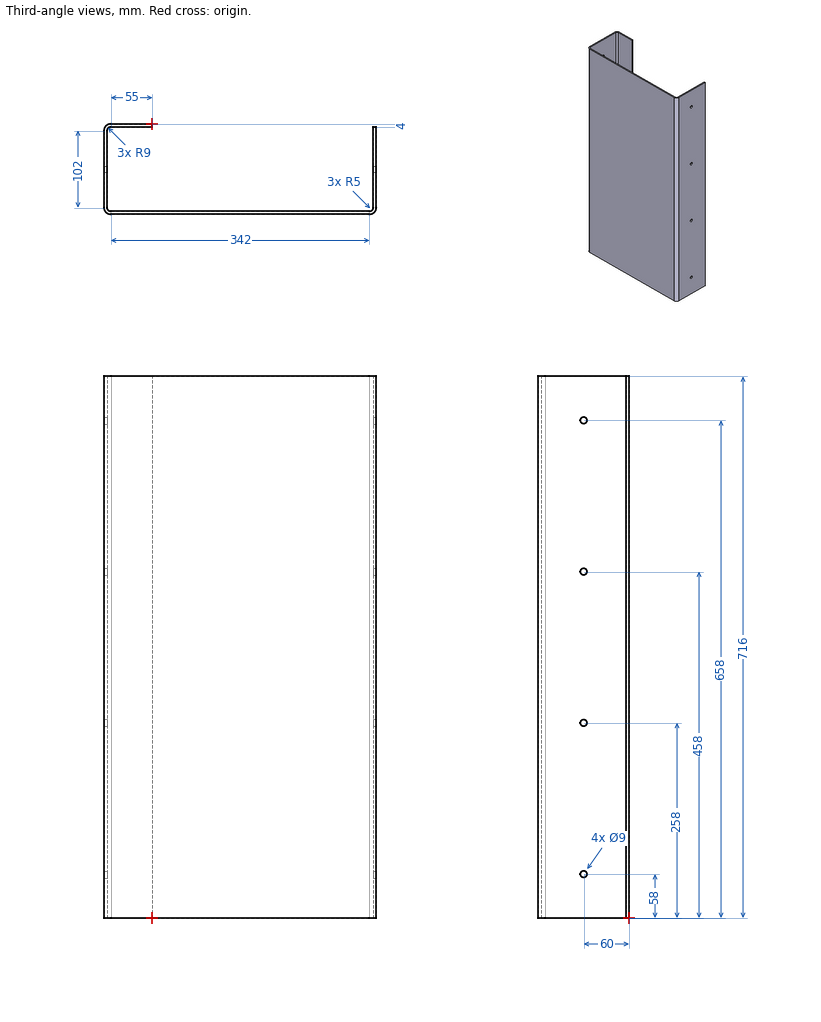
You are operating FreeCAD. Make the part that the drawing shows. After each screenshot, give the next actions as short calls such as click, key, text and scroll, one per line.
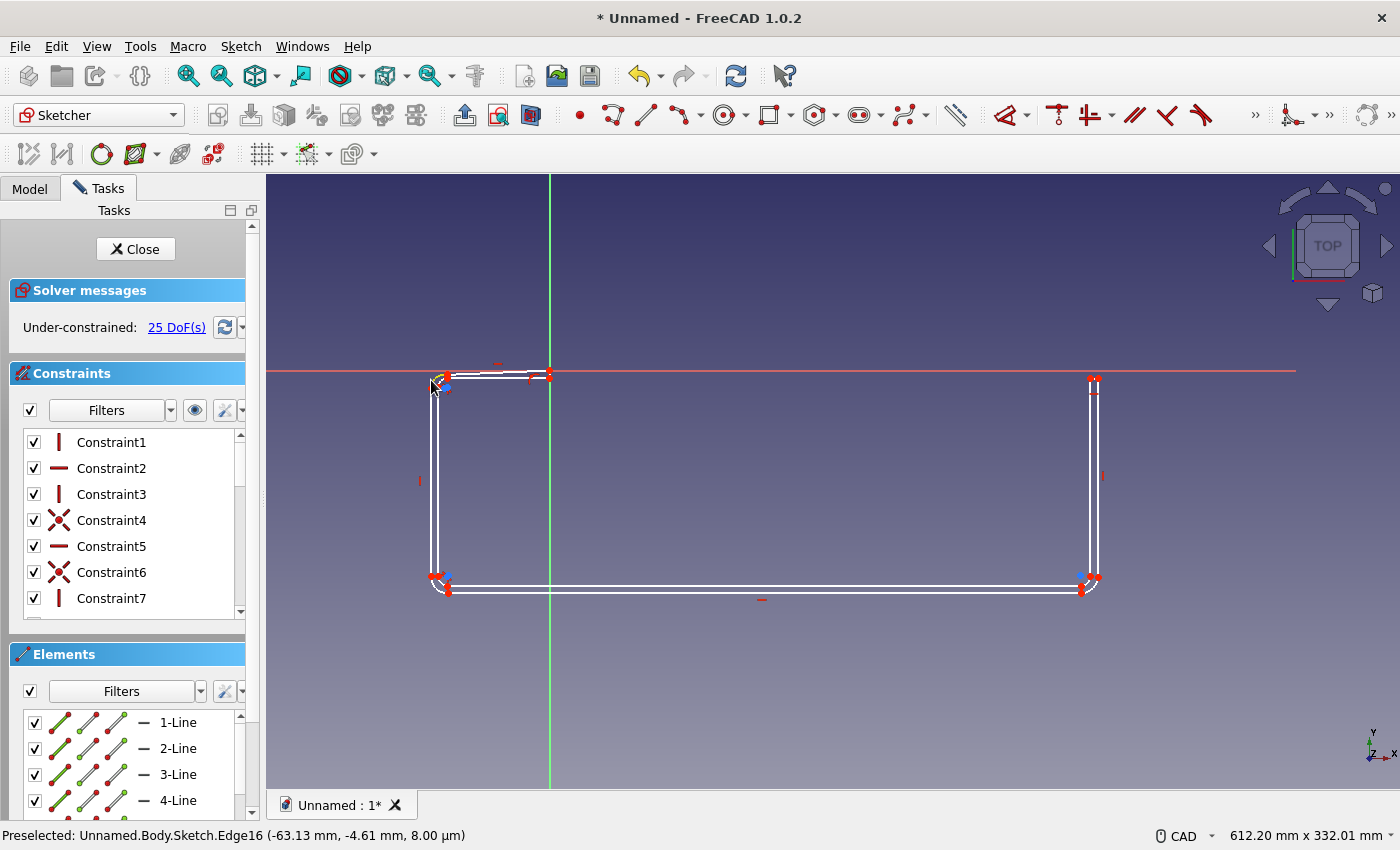
scroll(638, 593, up, 4)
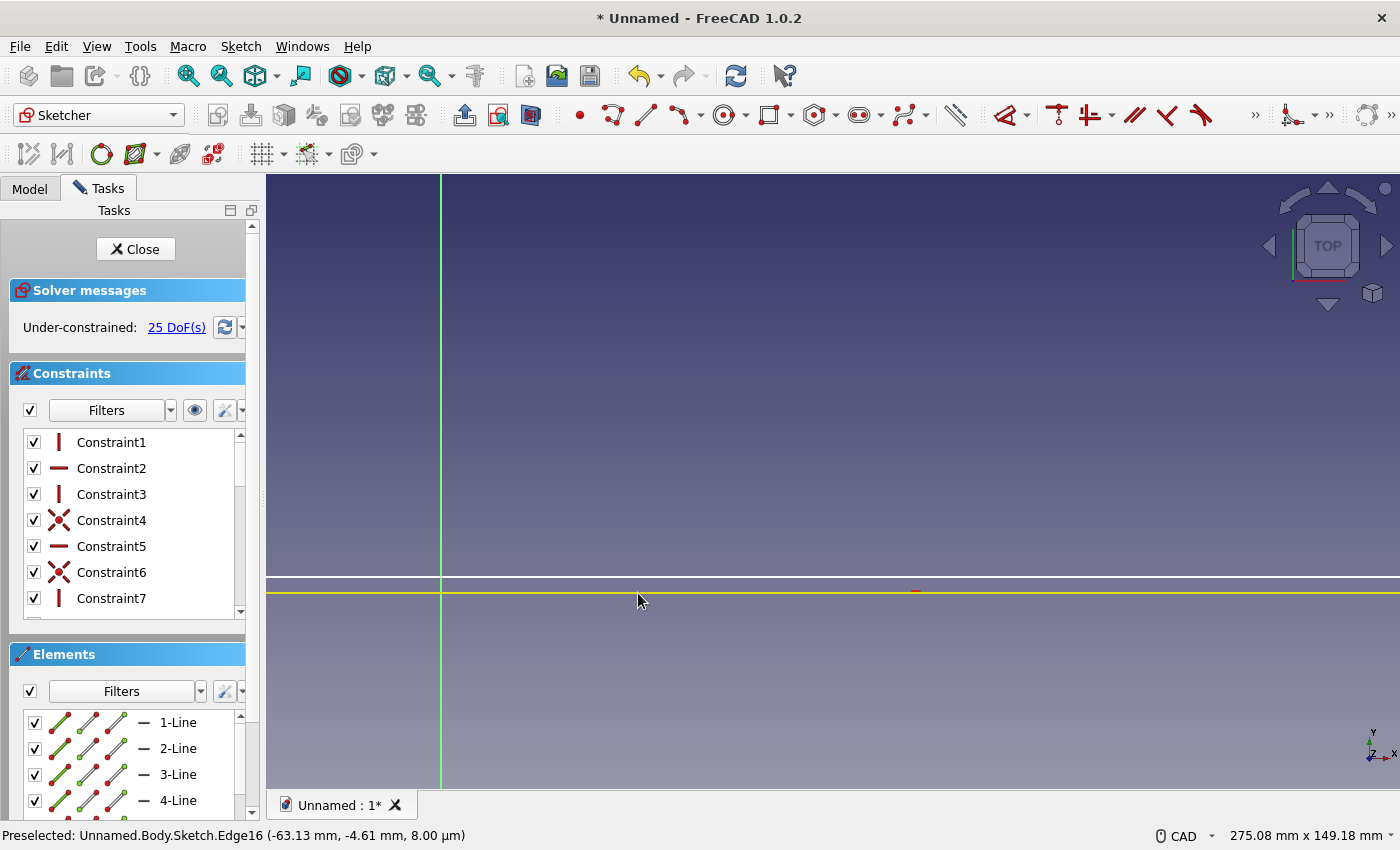
click(638, 593)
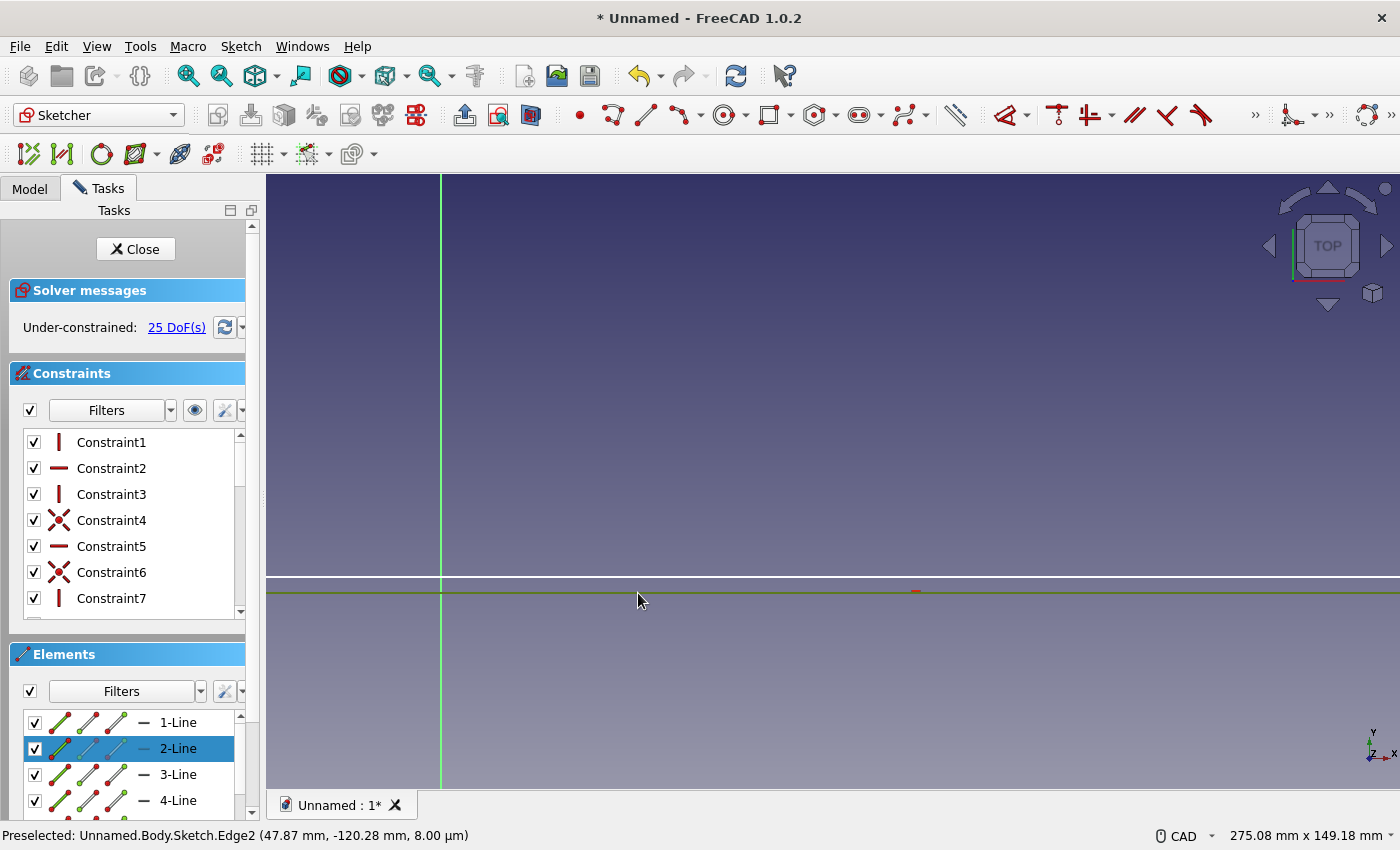
scroll(639, 593, down, 4)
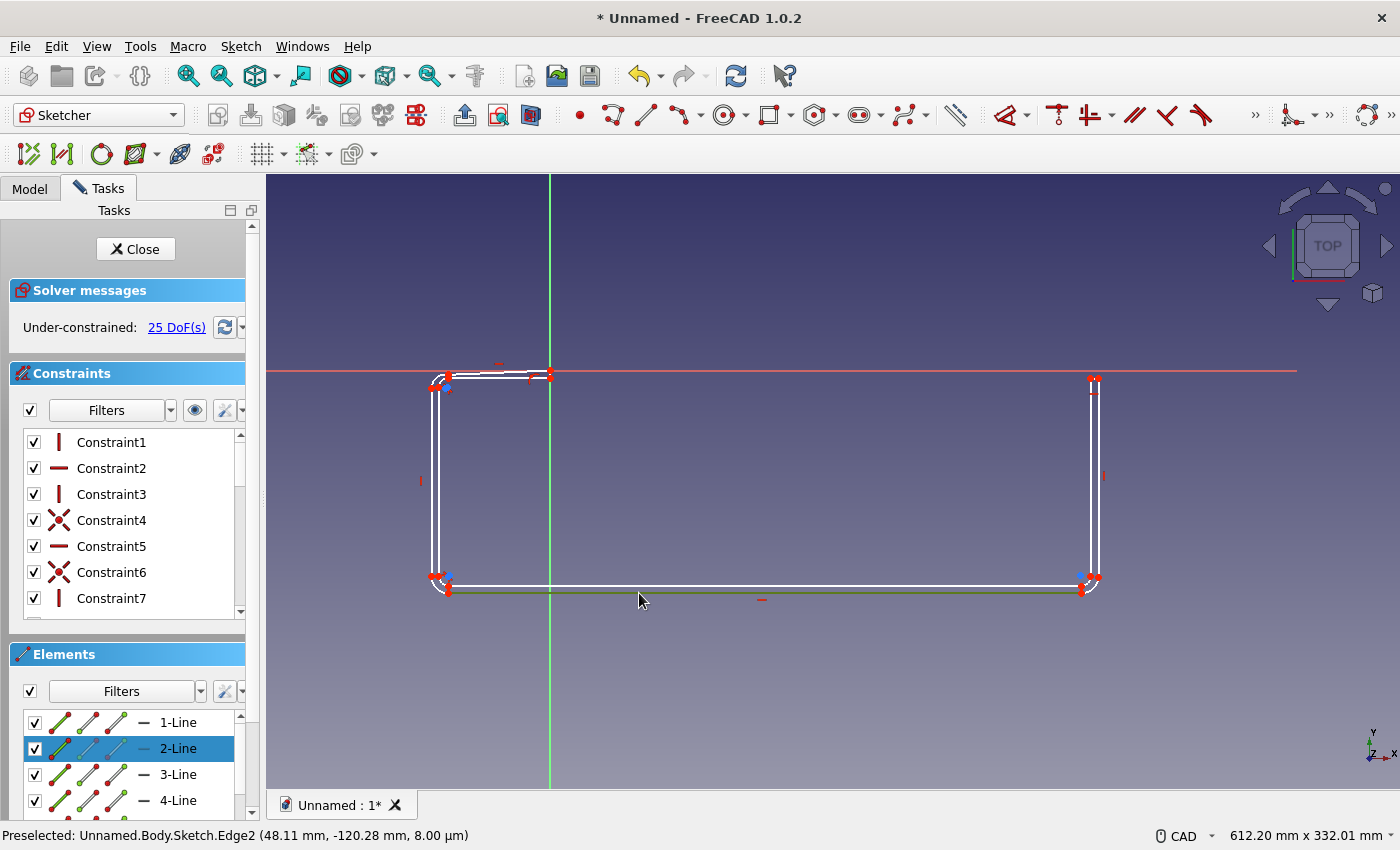
scroll(434, 584, up, 4)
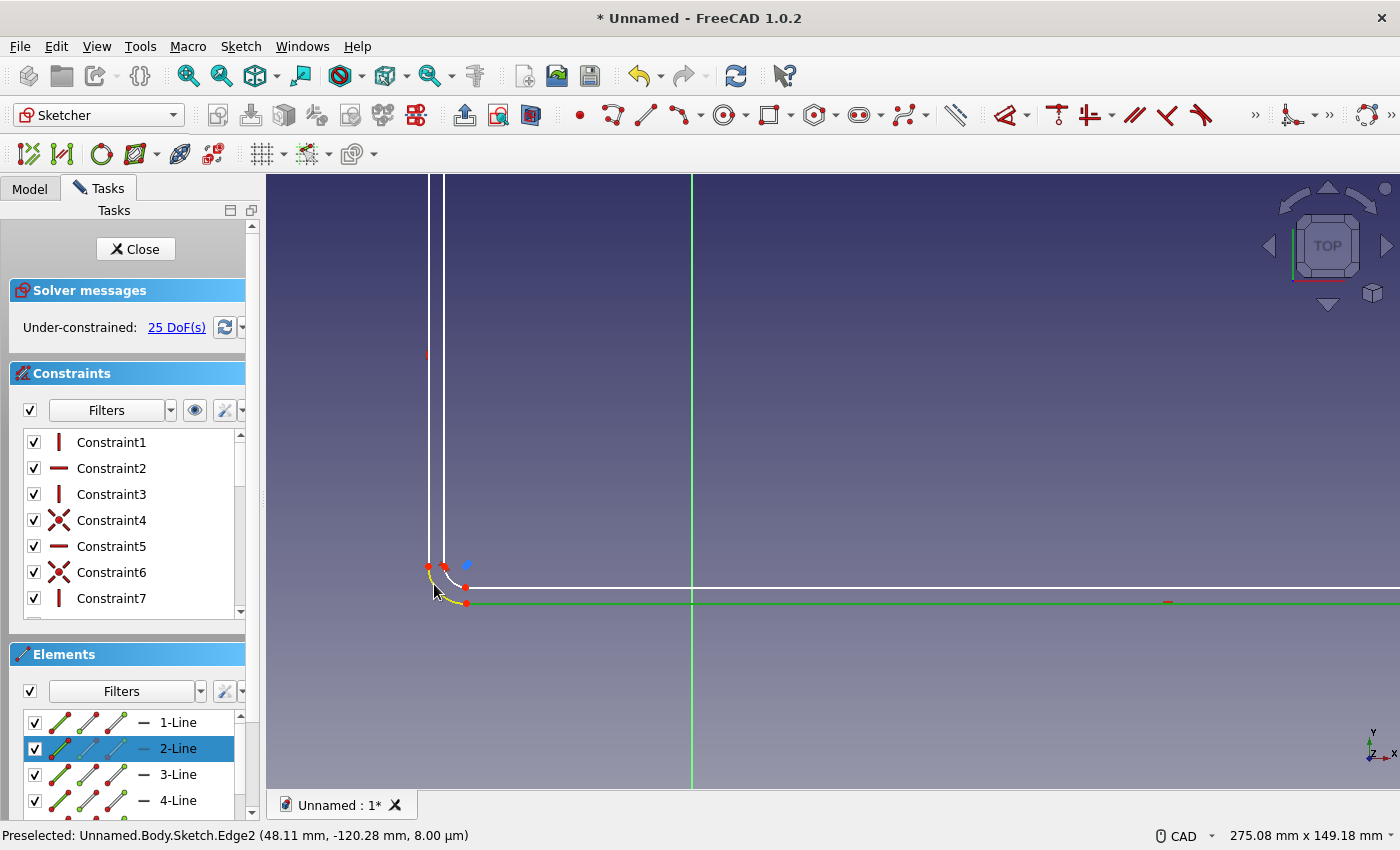
click(433, 584)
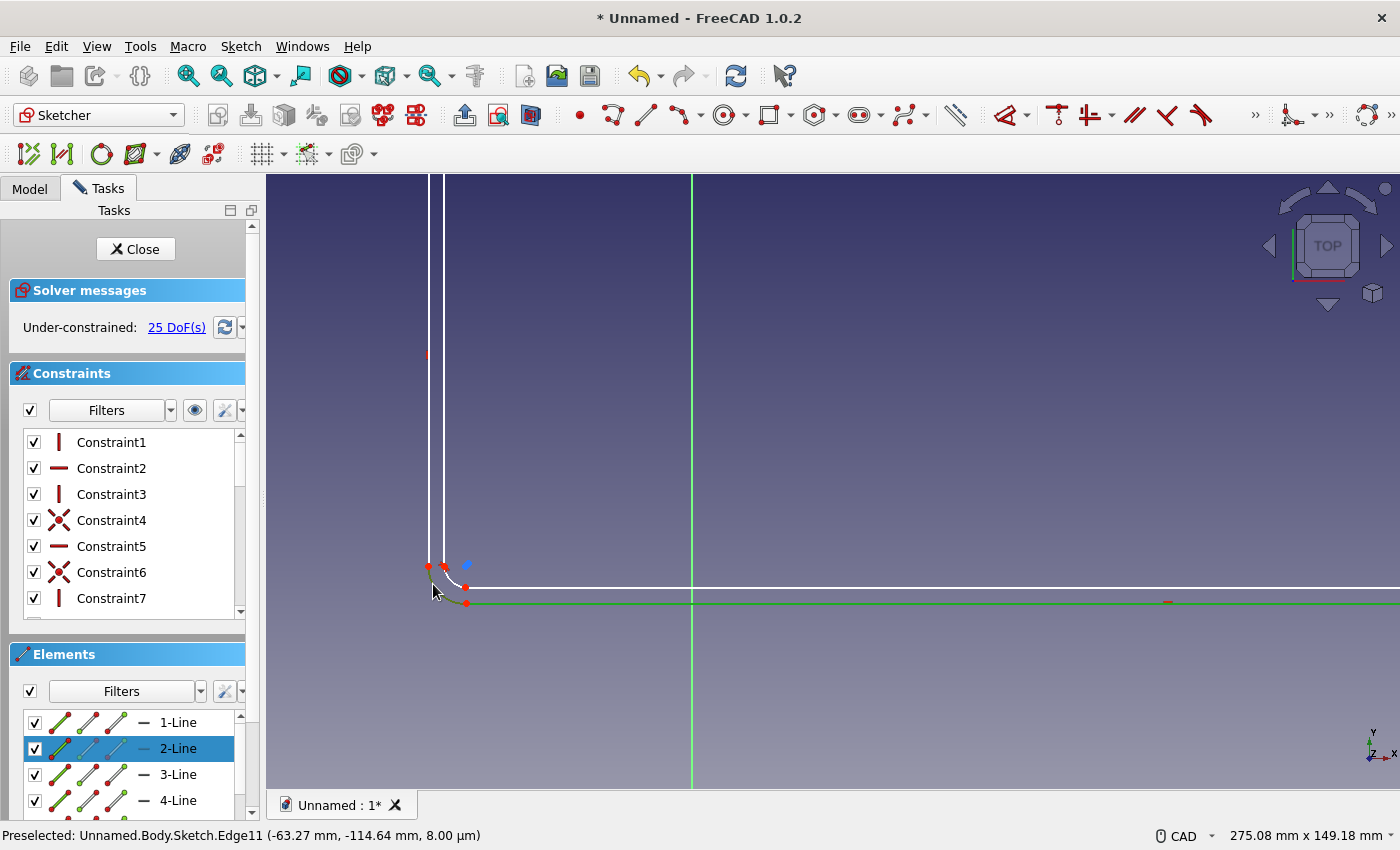
click(1201, 116)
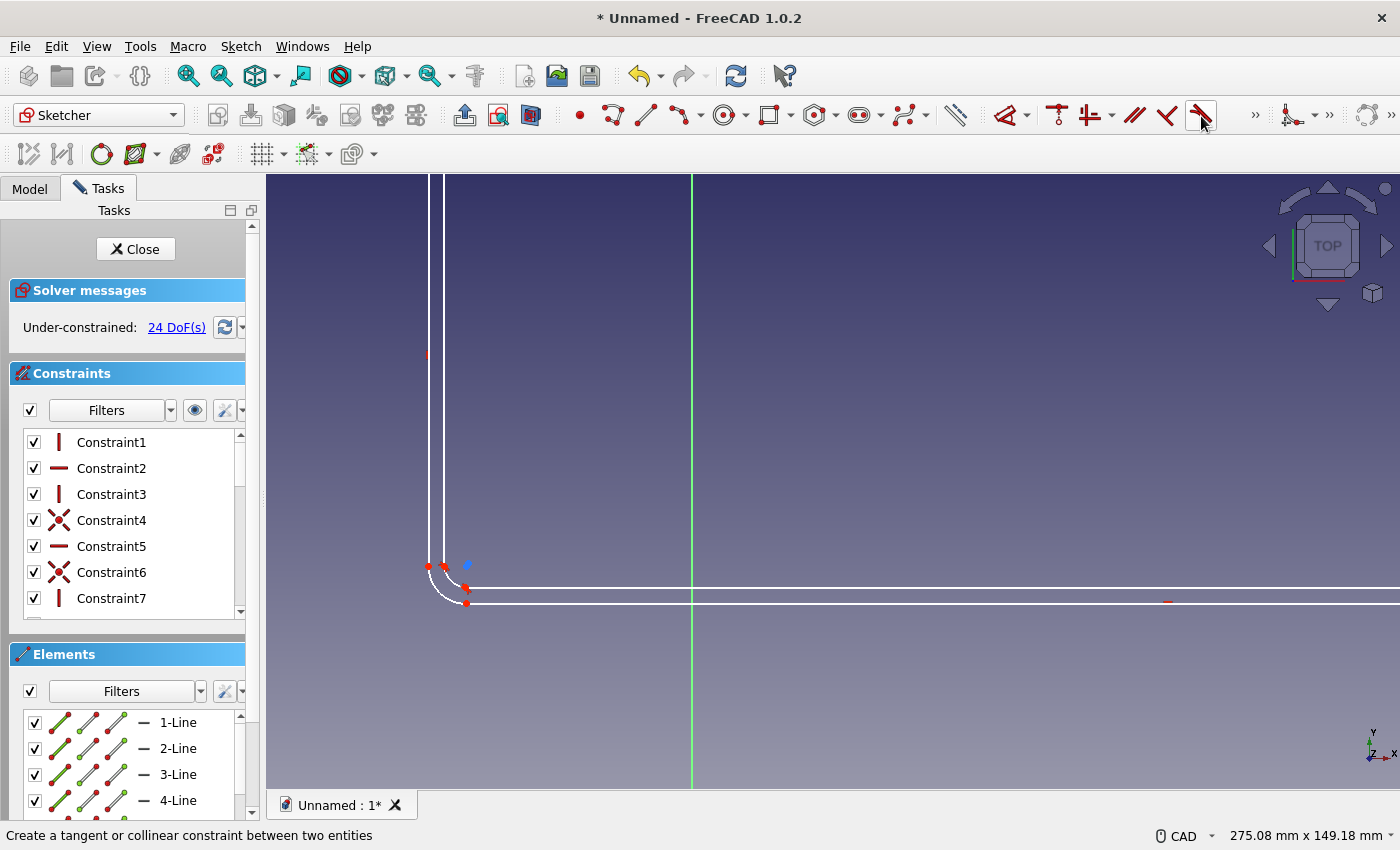
click(889, 604)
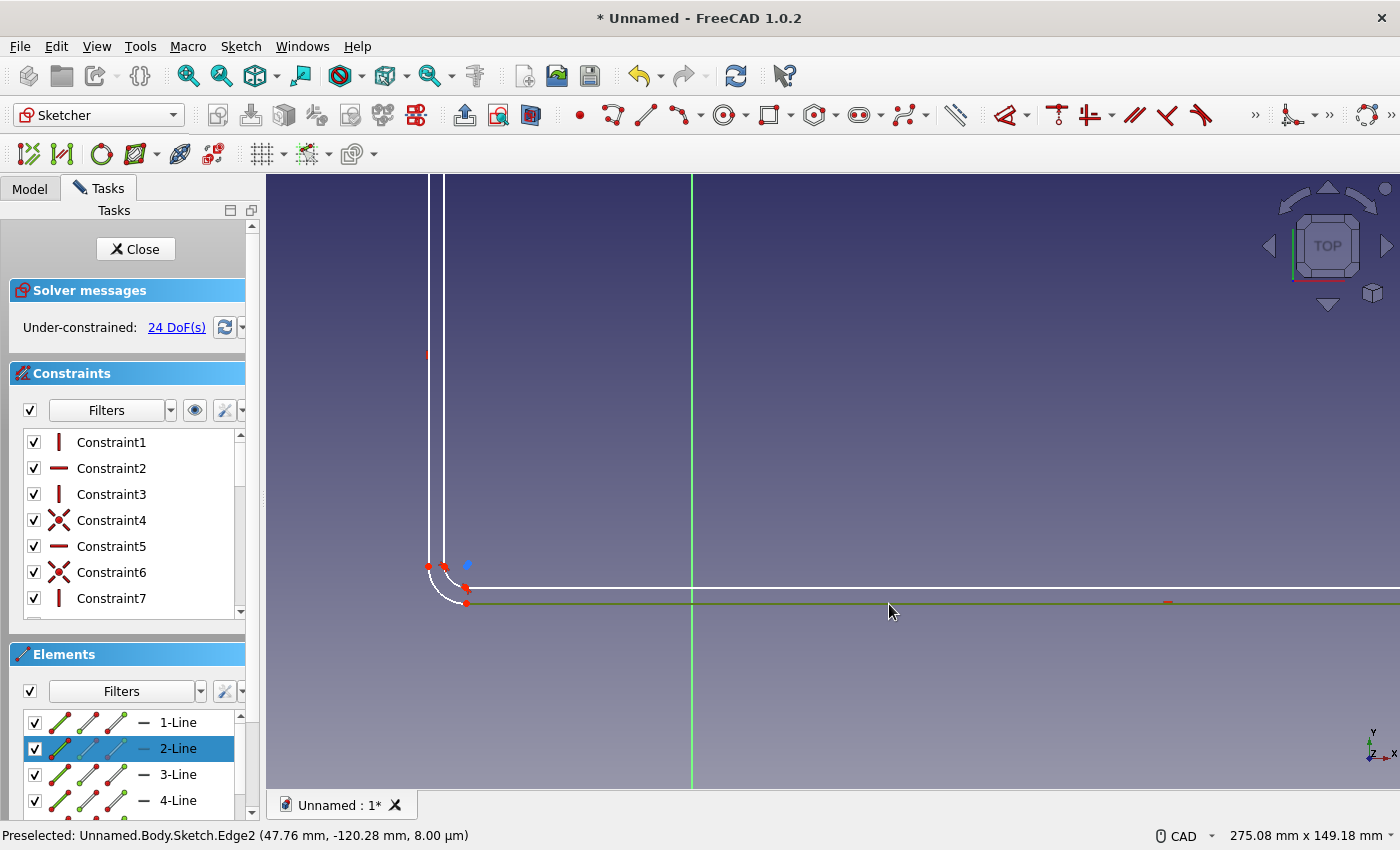
scroll(433, 584, down, 4)